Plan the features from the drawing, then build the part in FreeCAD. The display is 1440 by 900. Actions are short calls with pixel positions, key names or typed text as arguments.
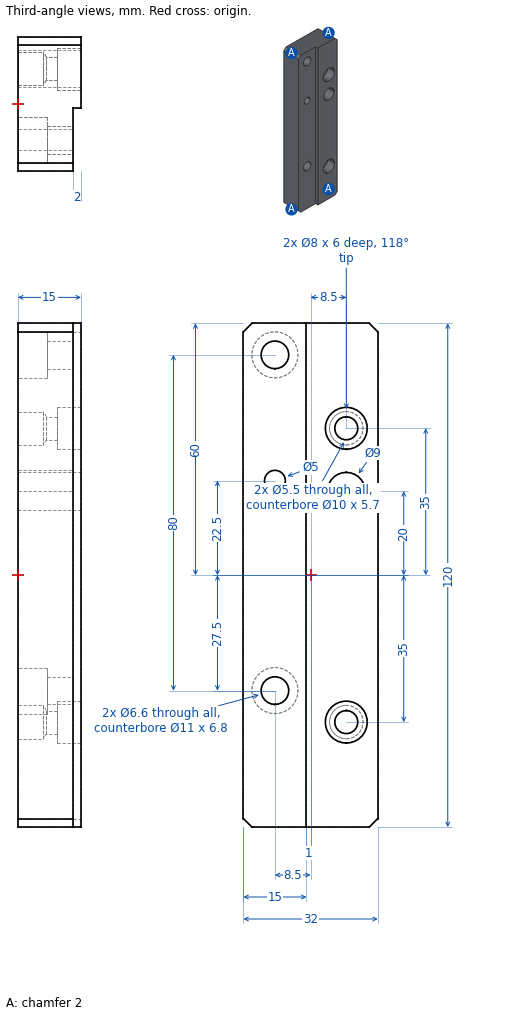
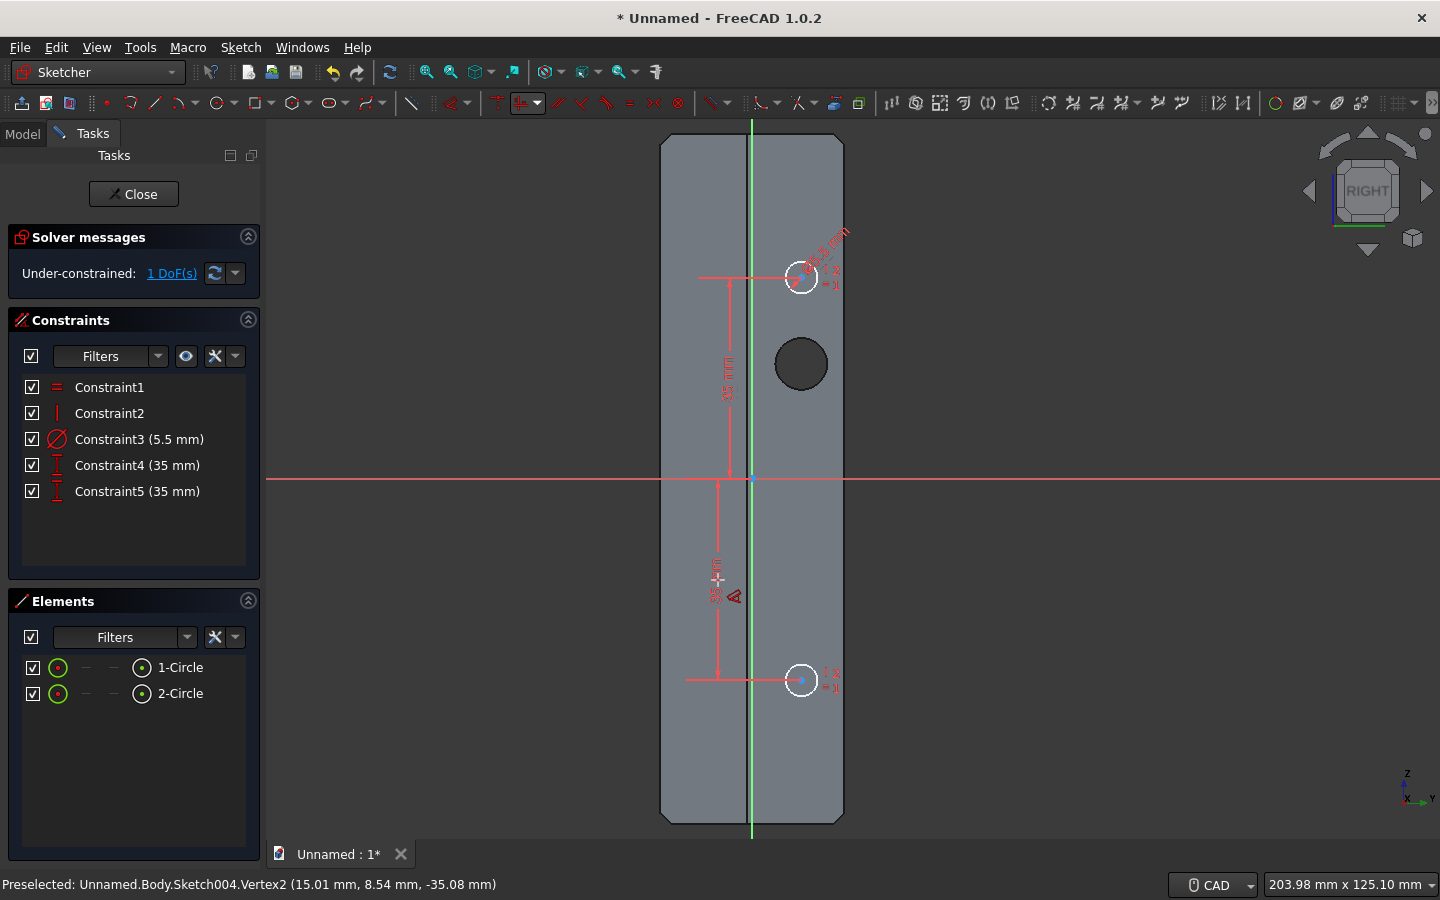
click(802, 278)
click(777, 513)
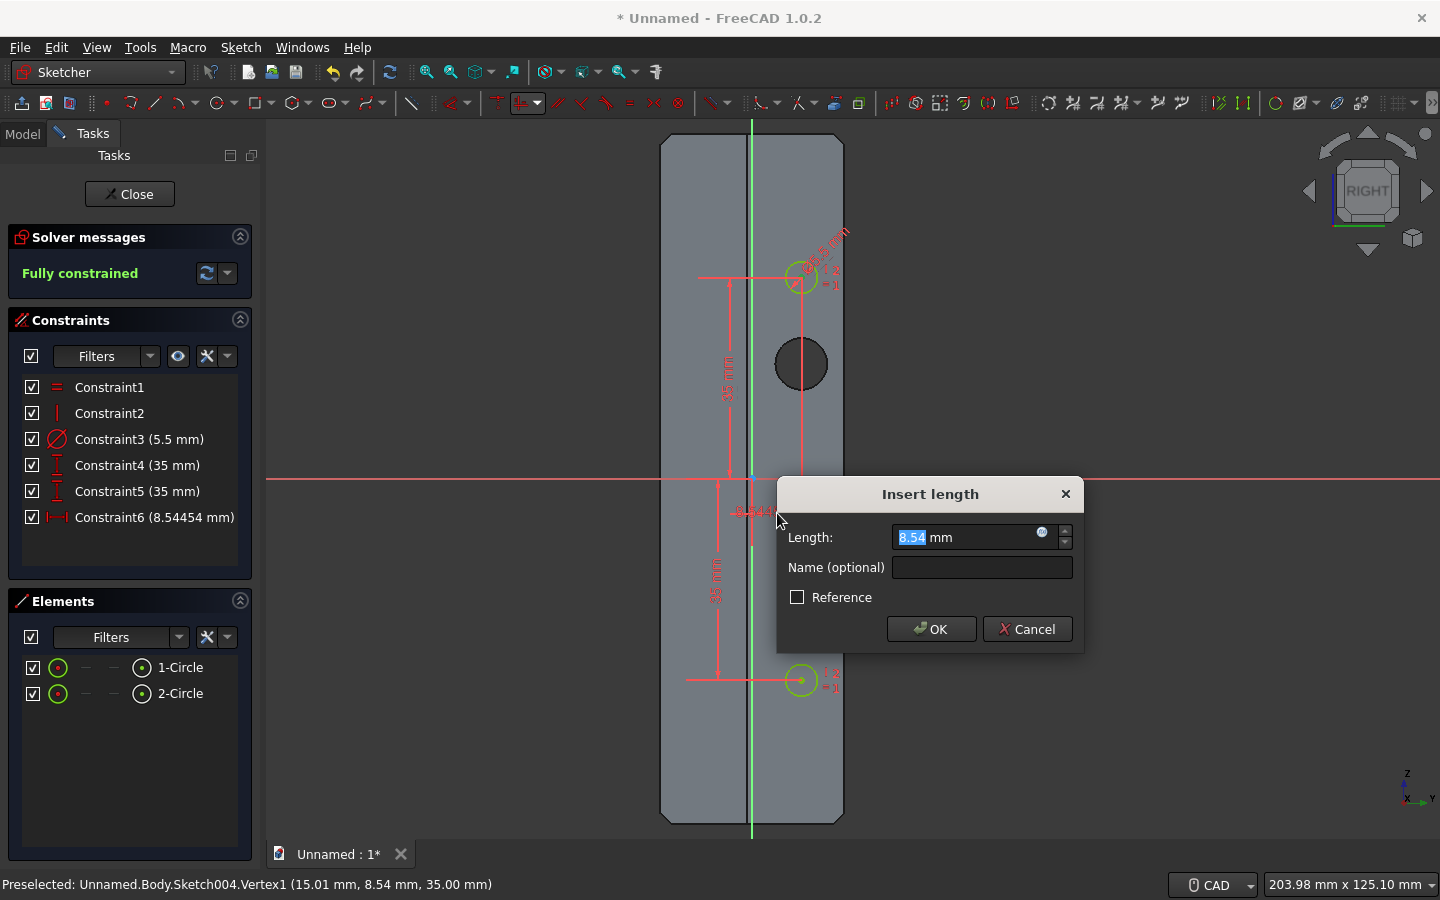
text(8.5)
key(Return)
key(Escape)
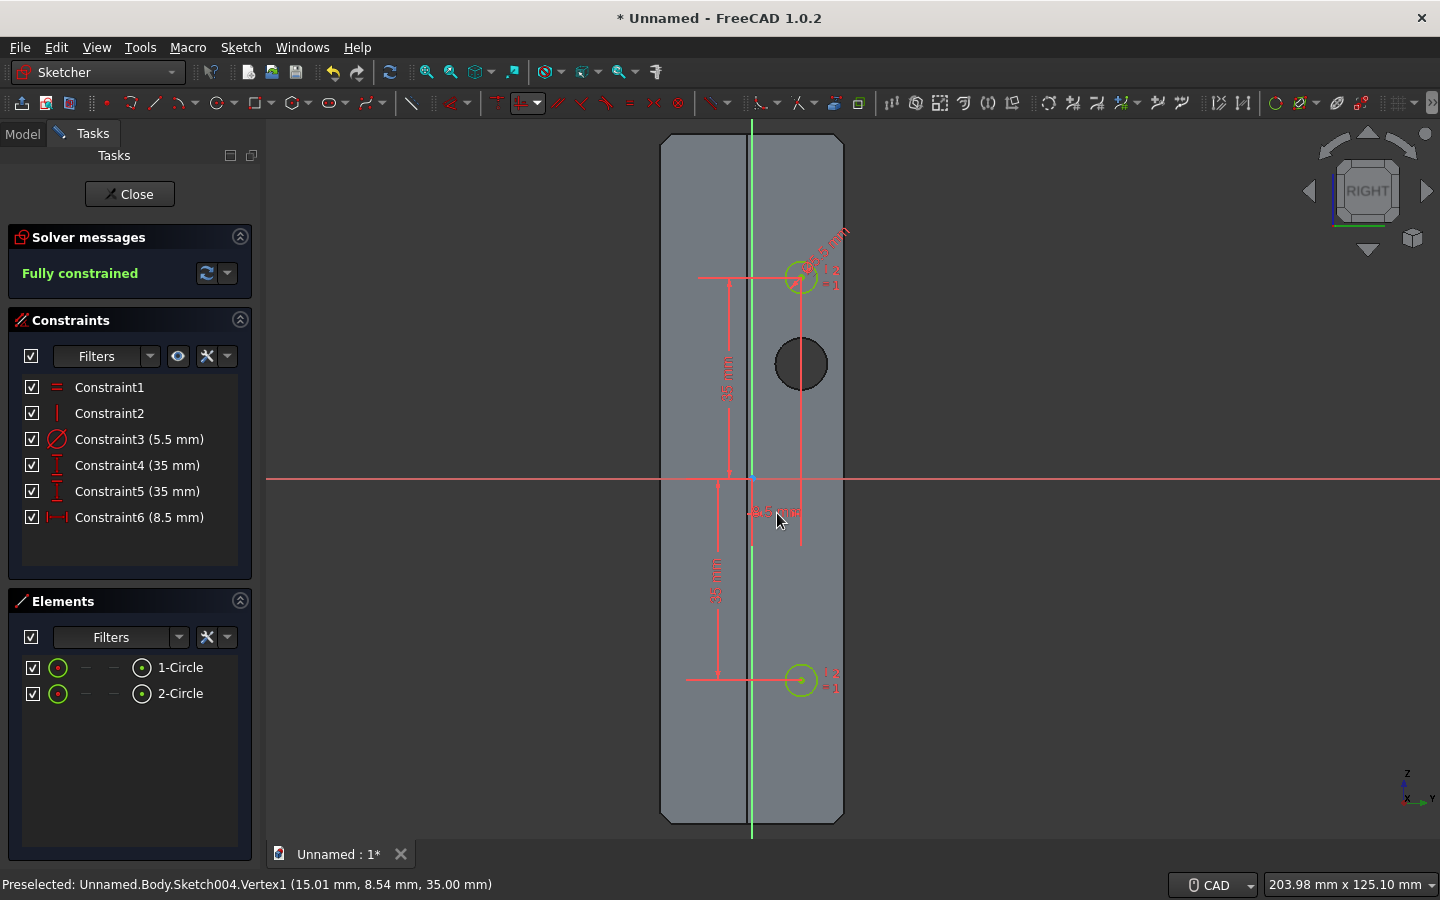
click(130, 194)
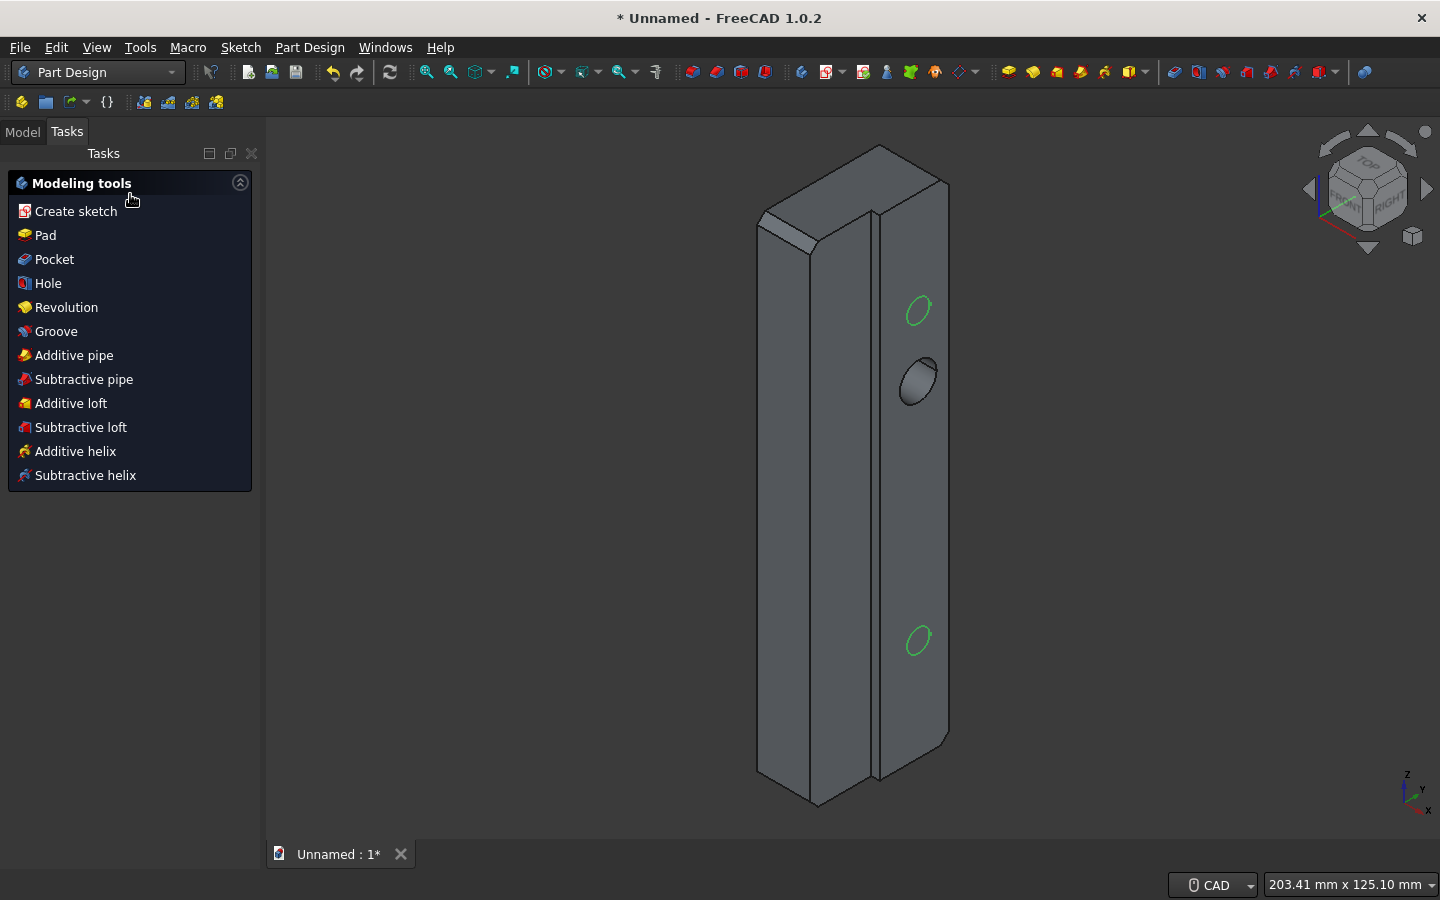
click(1200, 72)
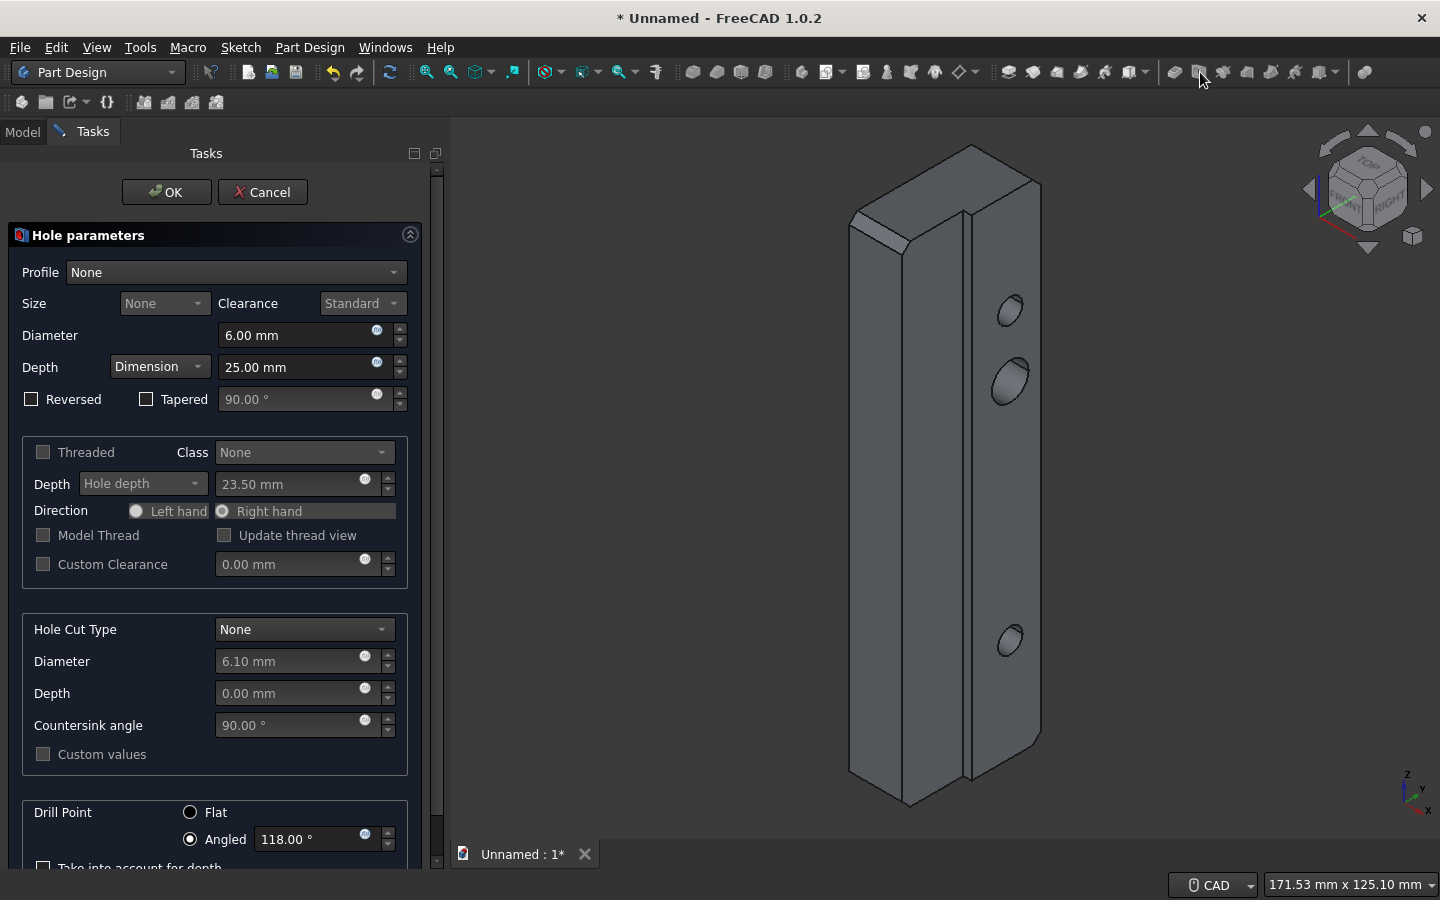
triple_click(305, 335)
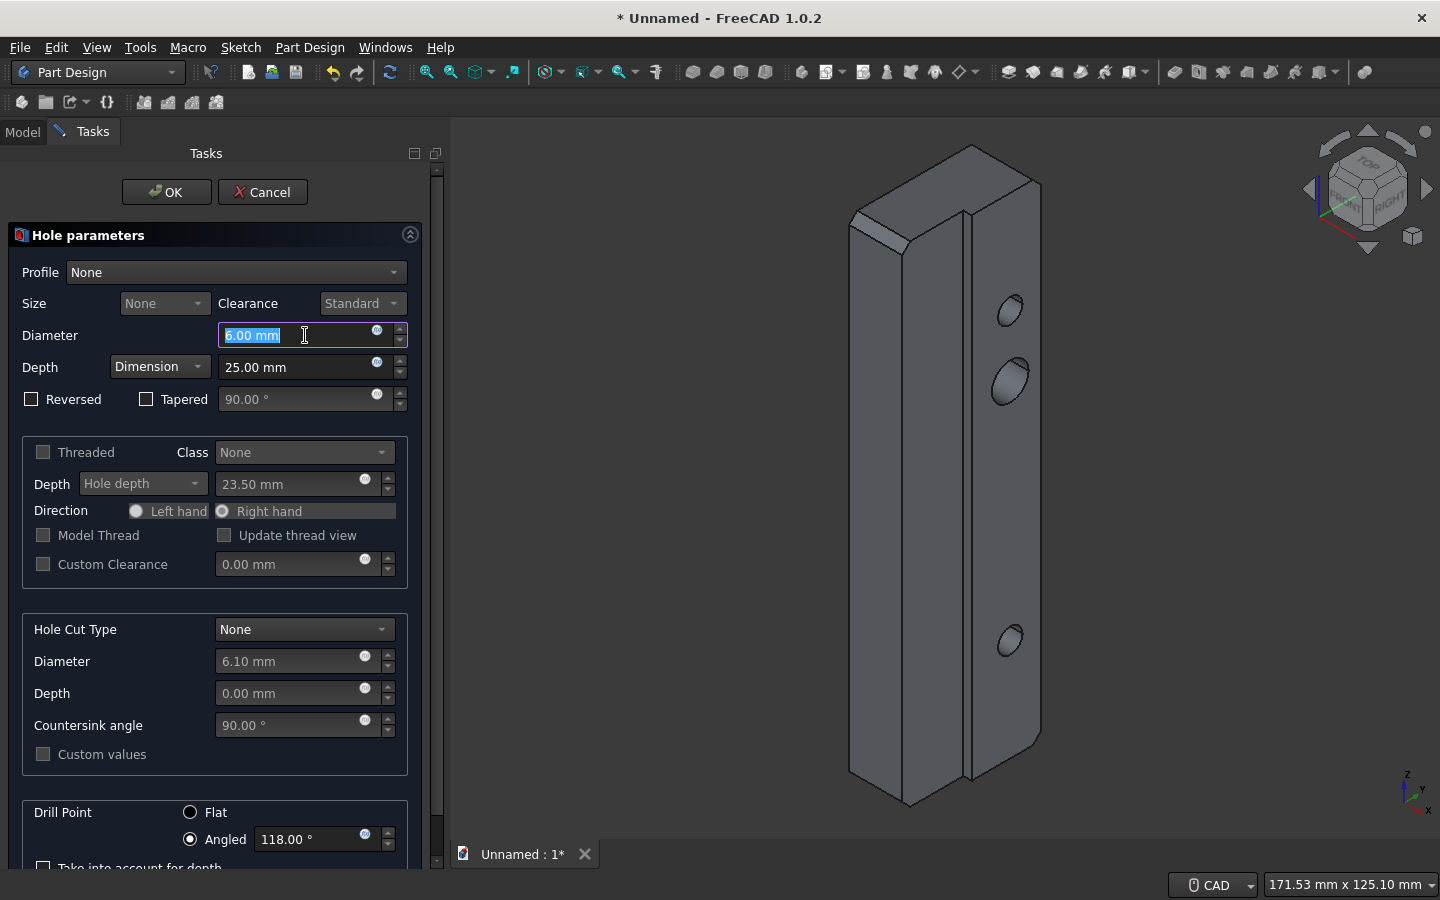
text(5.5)
key(Tab)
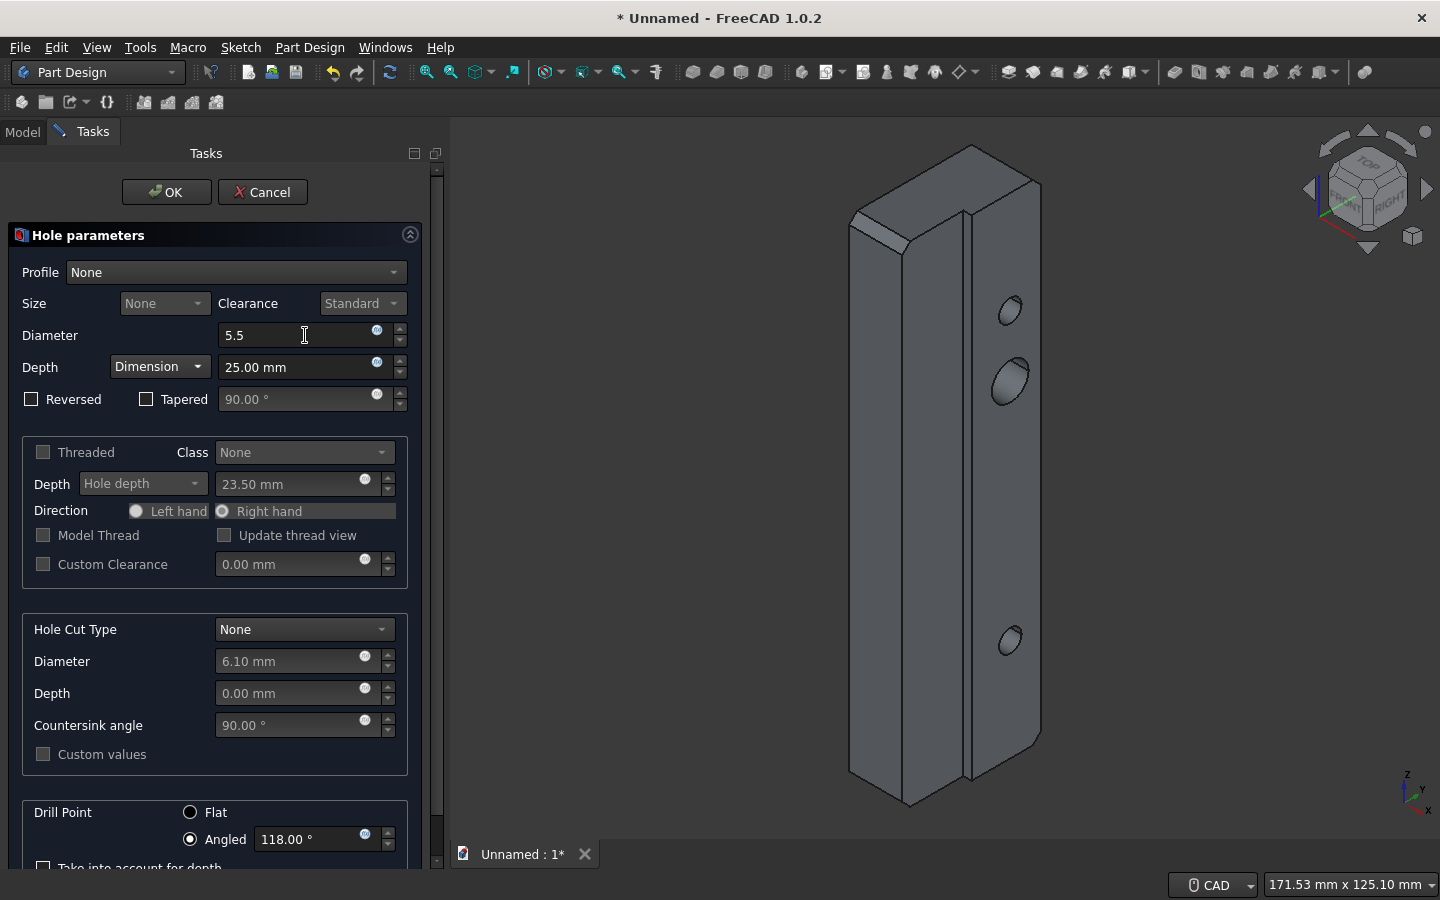
click(161, 366)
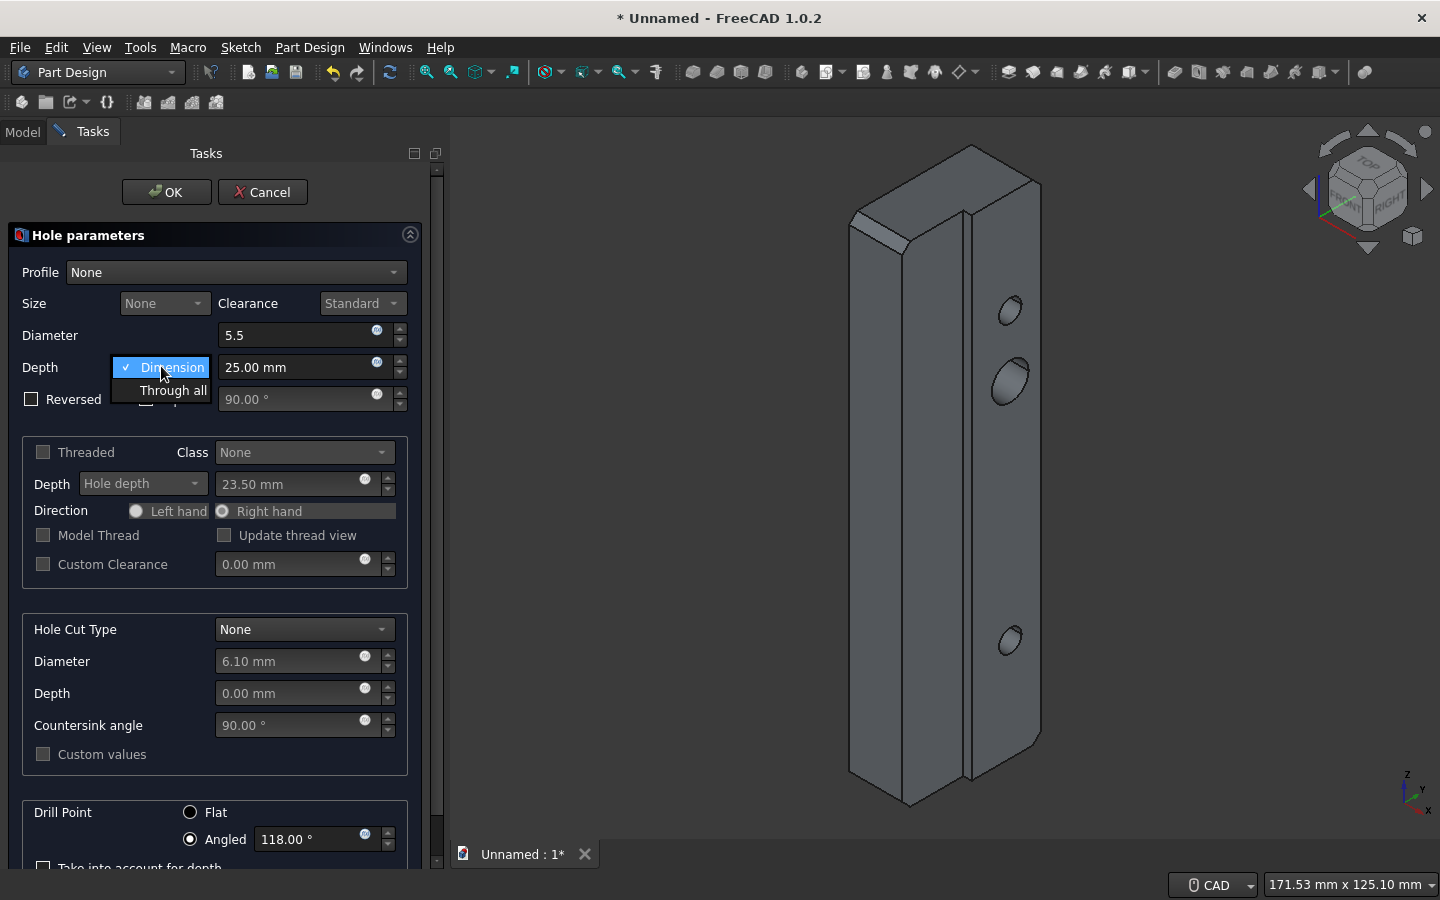
click(160, 390)